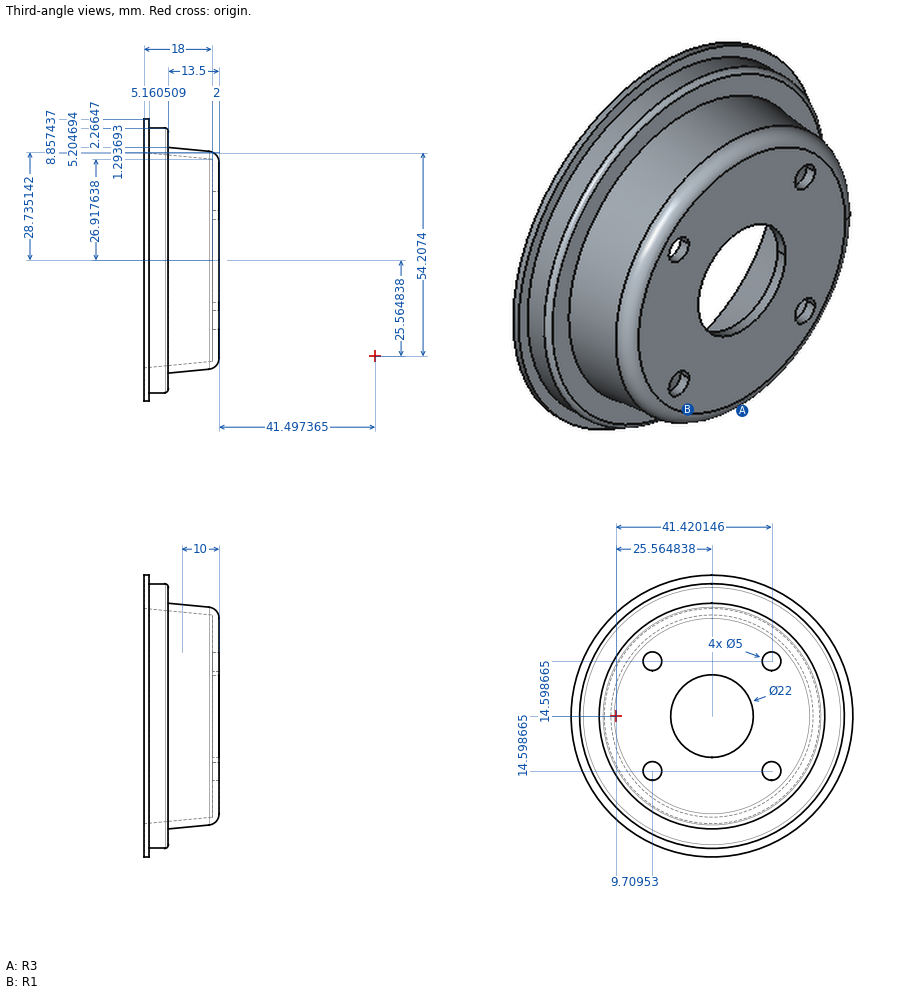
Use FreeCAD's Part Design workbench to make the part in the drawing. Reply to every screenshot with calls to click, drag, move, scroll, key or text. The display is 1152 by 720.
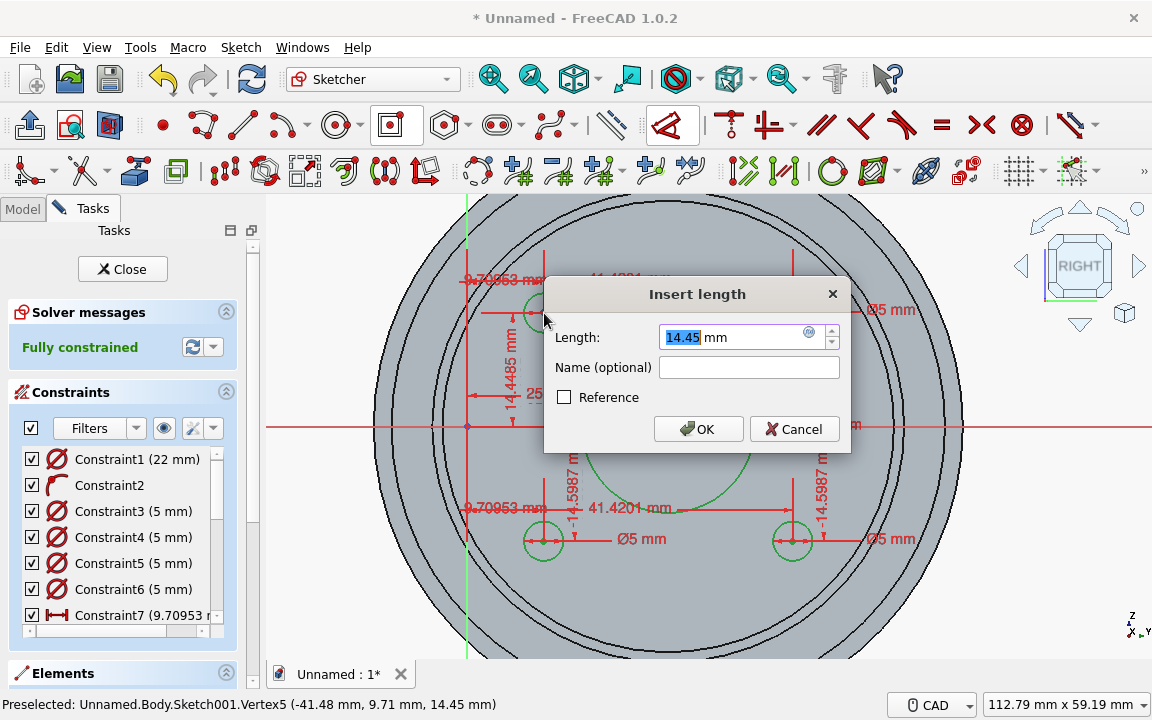
text(14.598665)
key(Return)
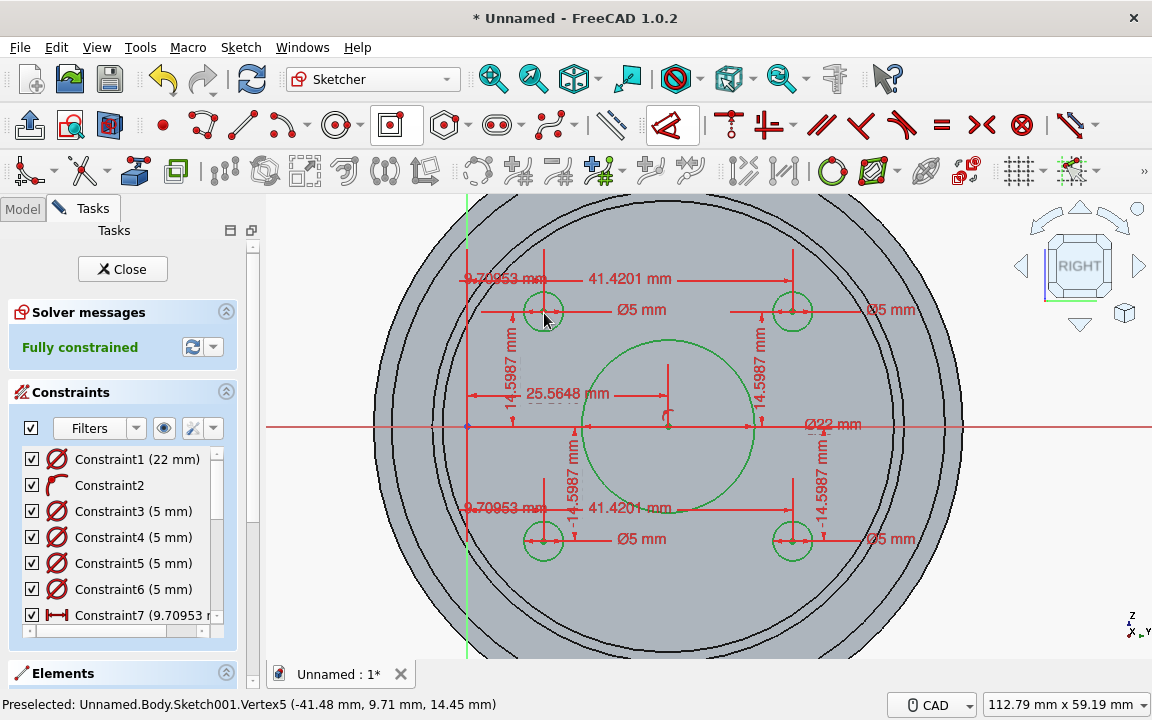
click(123, 269)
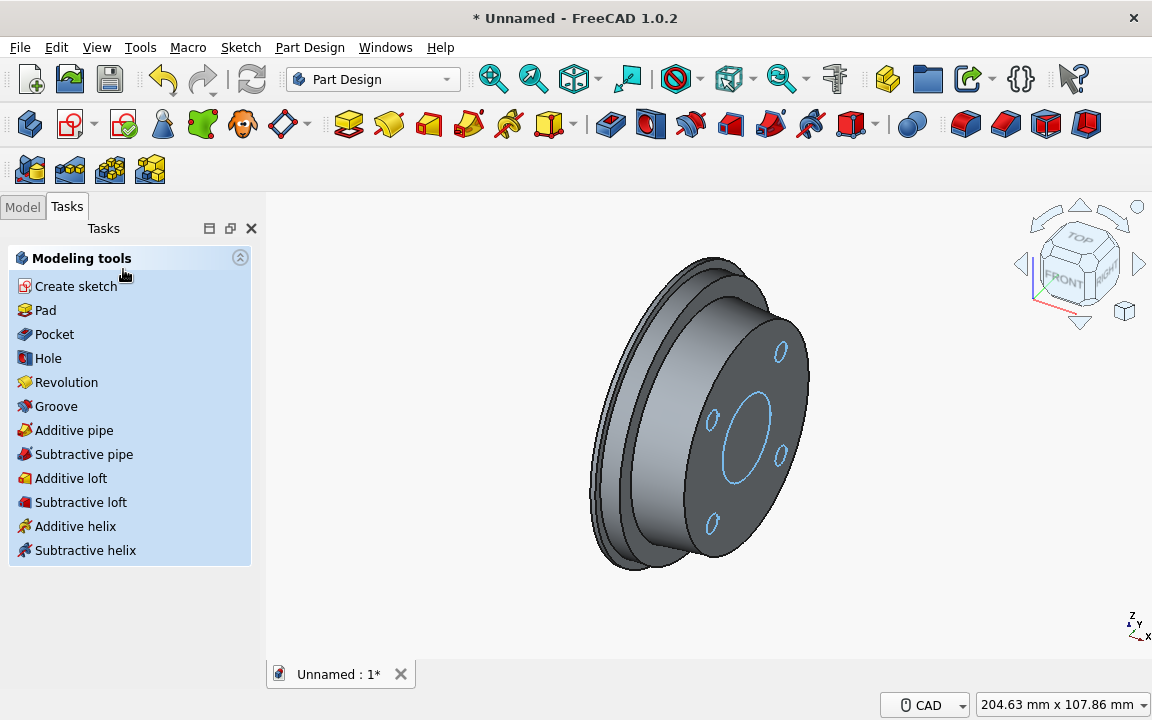
click(612, 124)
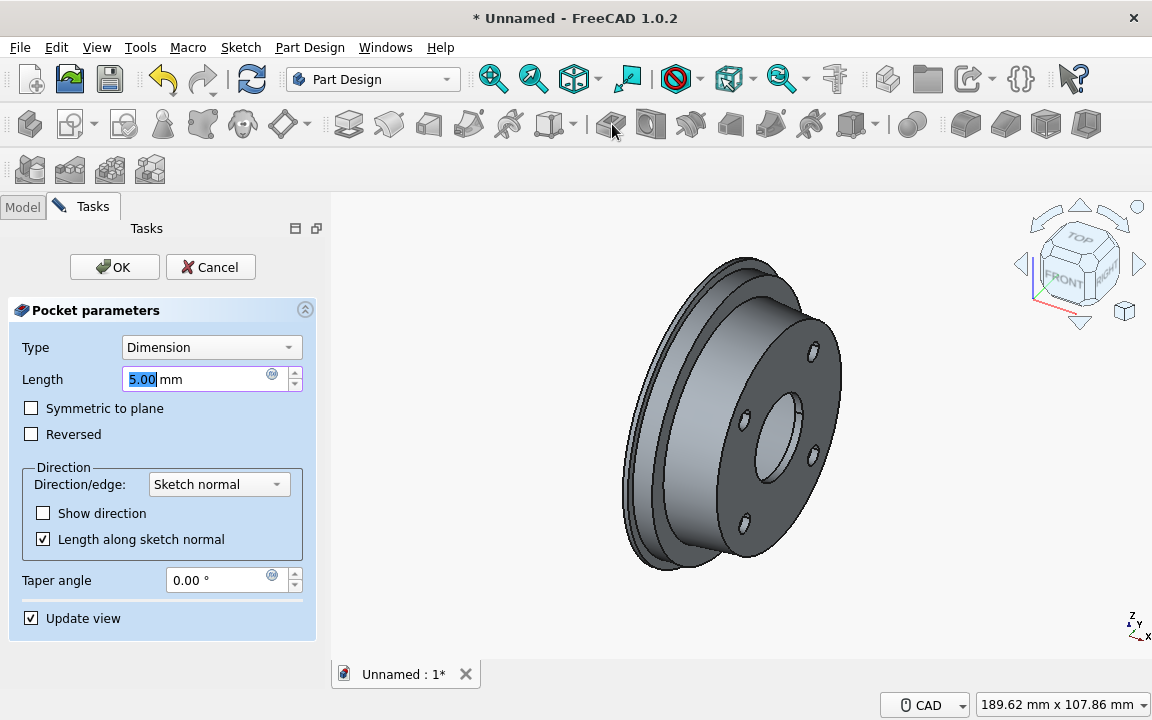
text(10)
key(Tab)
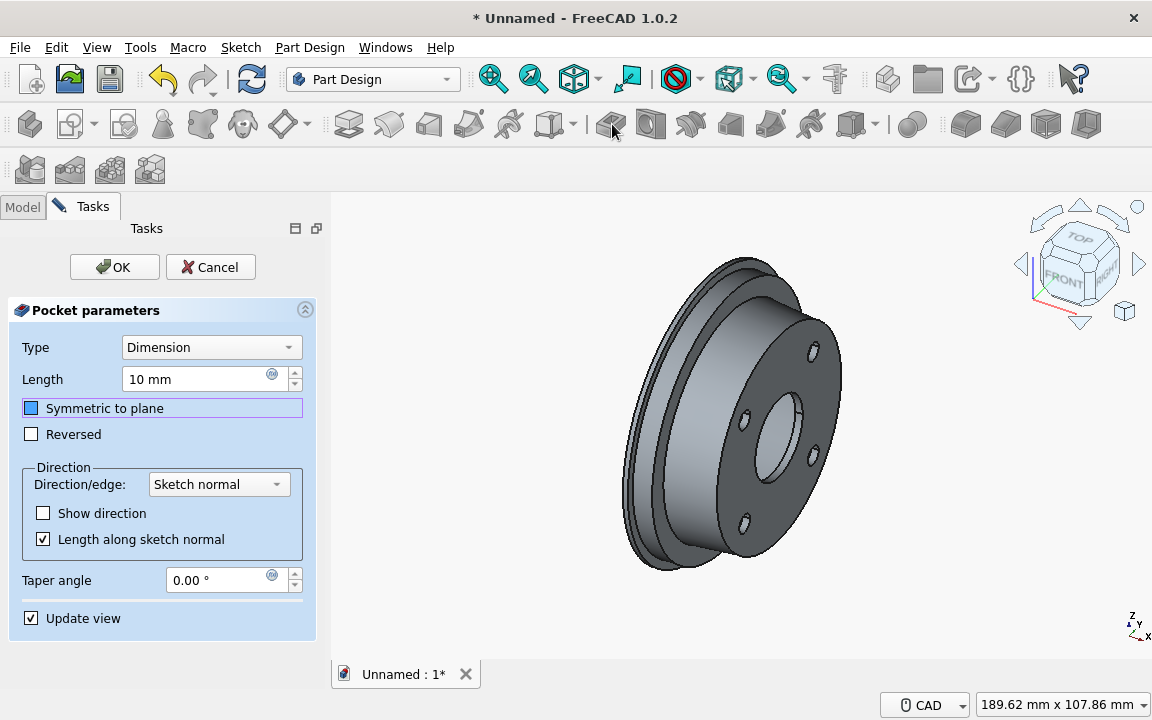
click(115, 267)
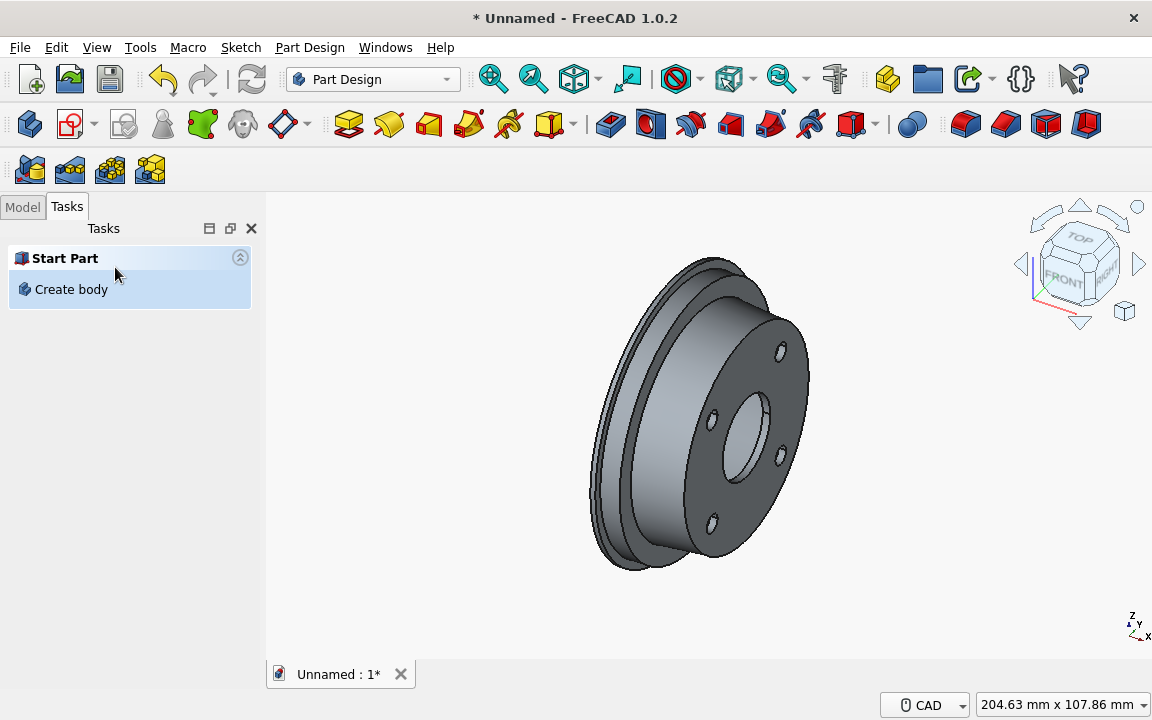
click(684, 499)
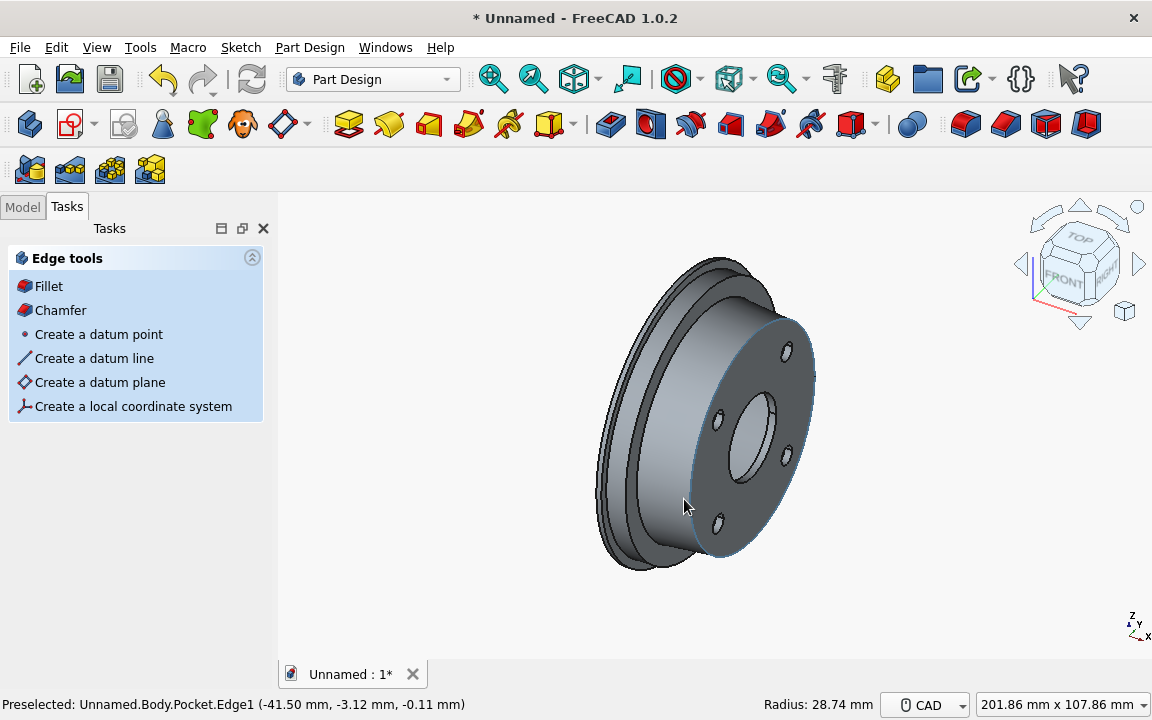
click(966, 124)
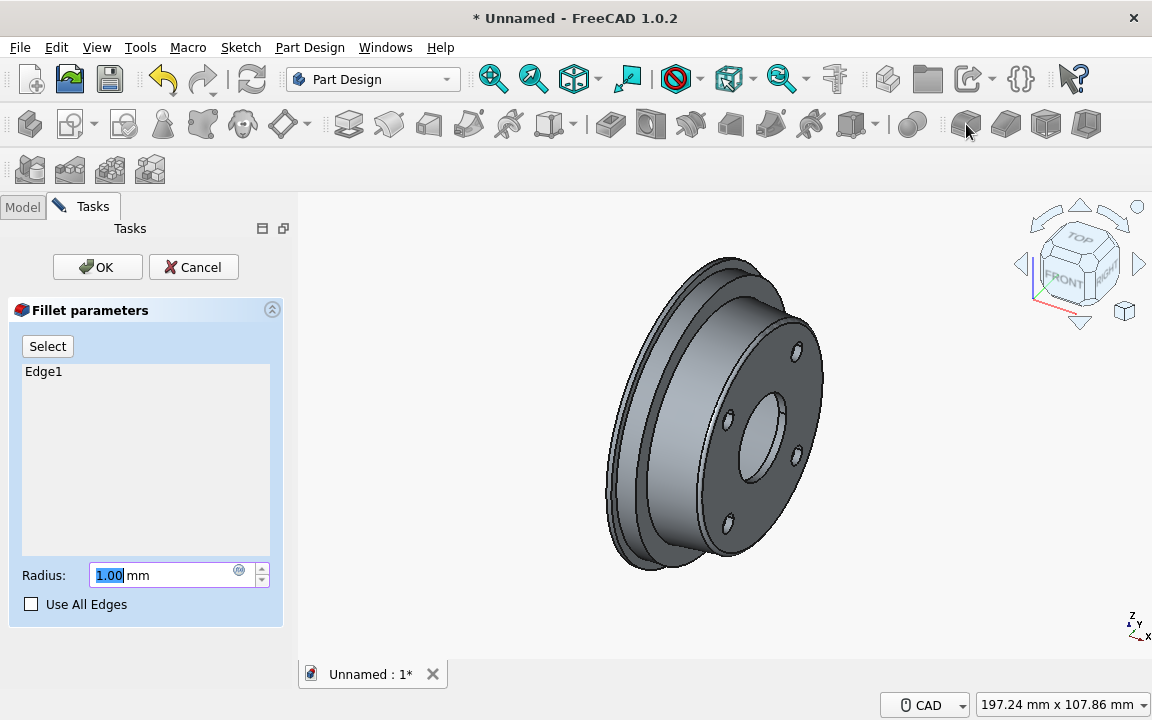
text(3)
key(Tab)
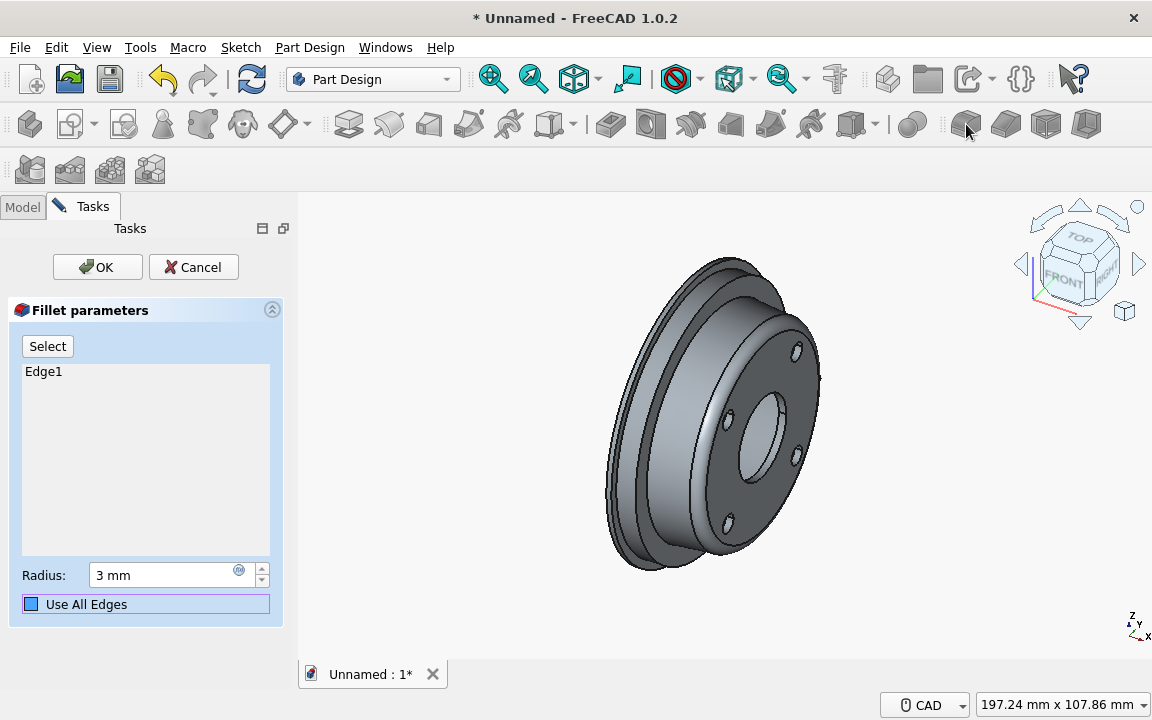
click(98, 267)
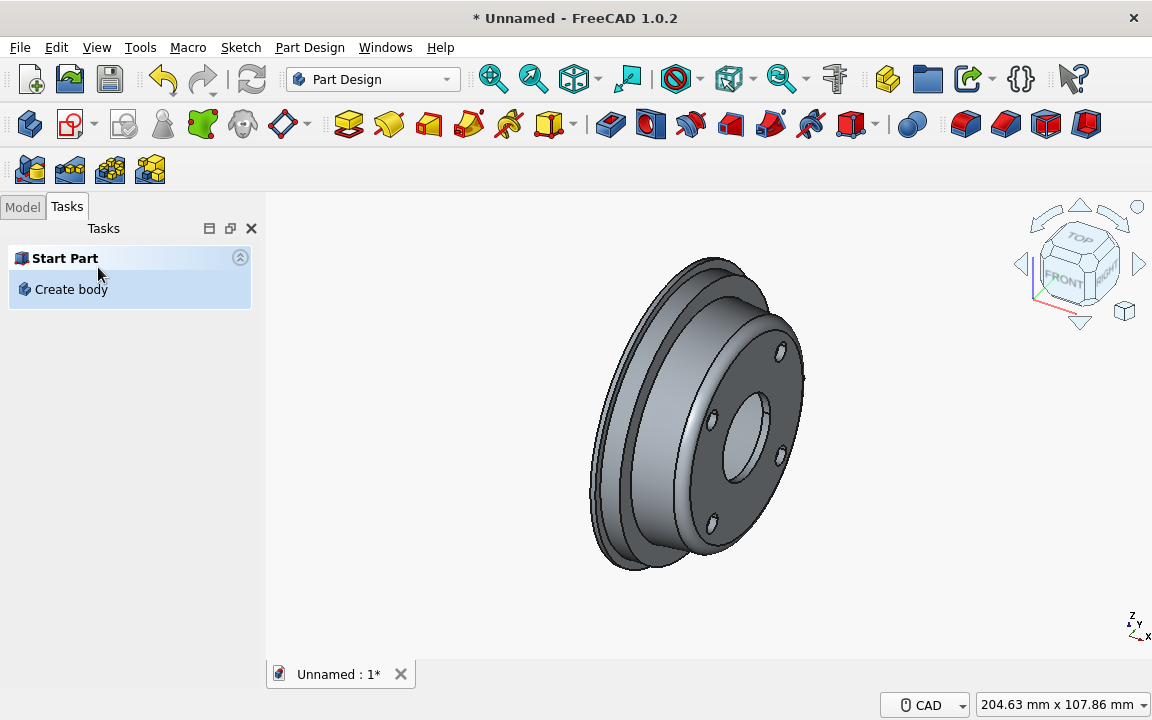
click(620, 496)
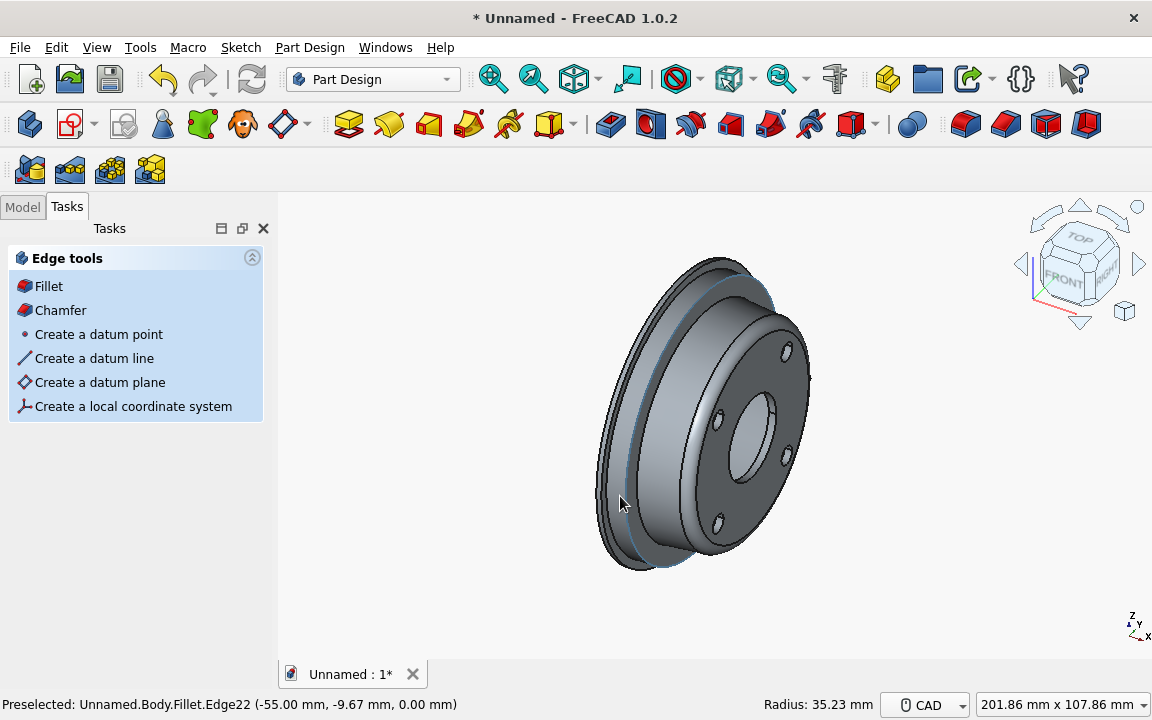
click(966, 124)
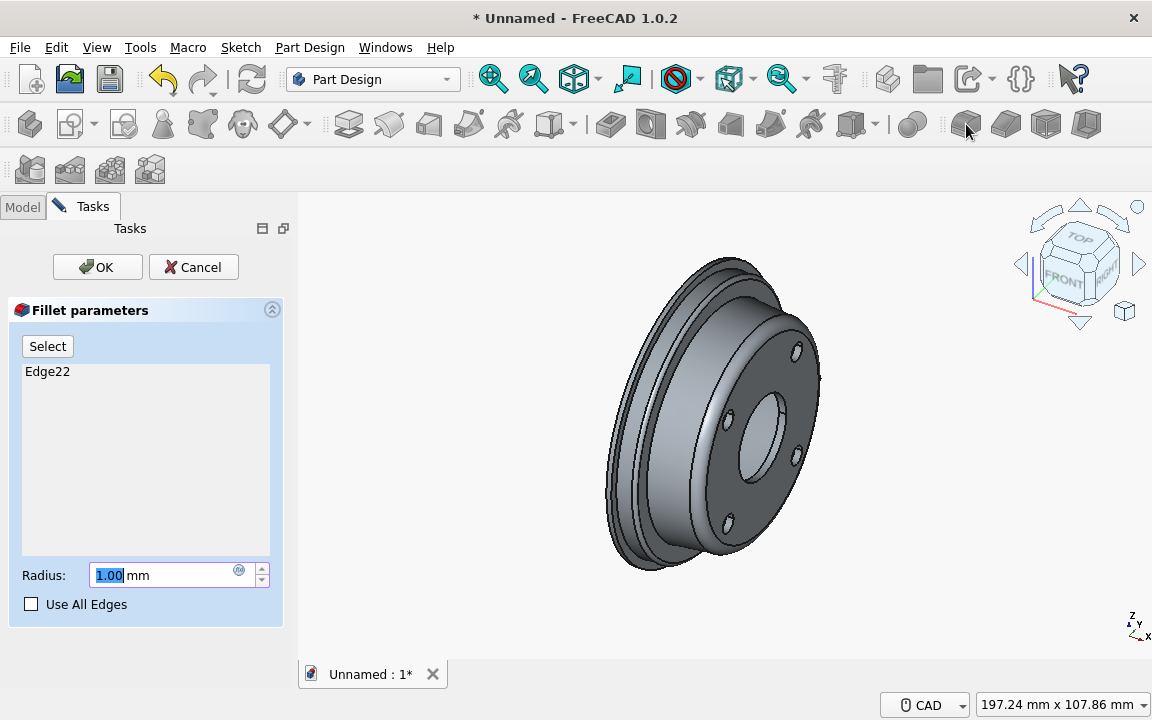
text(1)
key(Tab)